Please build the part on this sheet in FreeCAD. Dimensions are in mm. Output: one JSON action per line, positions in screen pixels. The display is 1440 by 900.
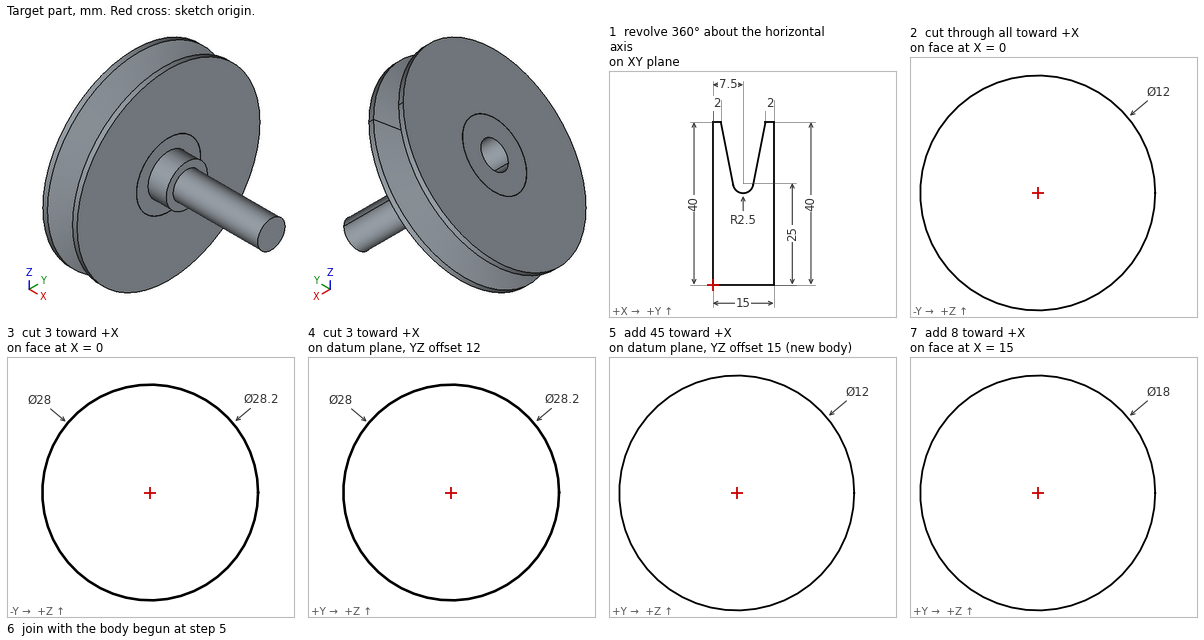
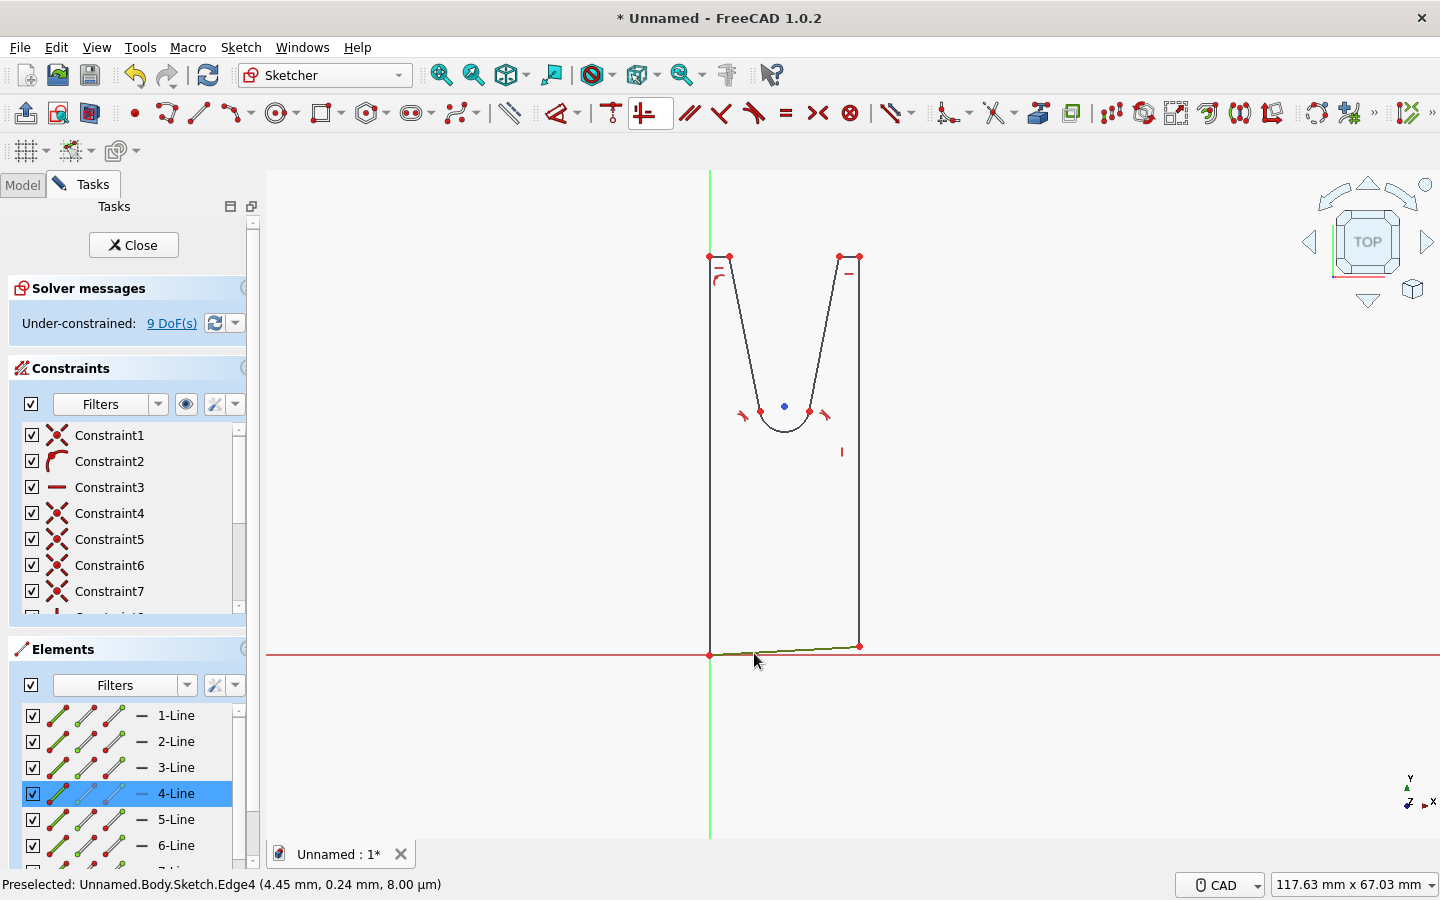
{"action": "key", "text": "h"}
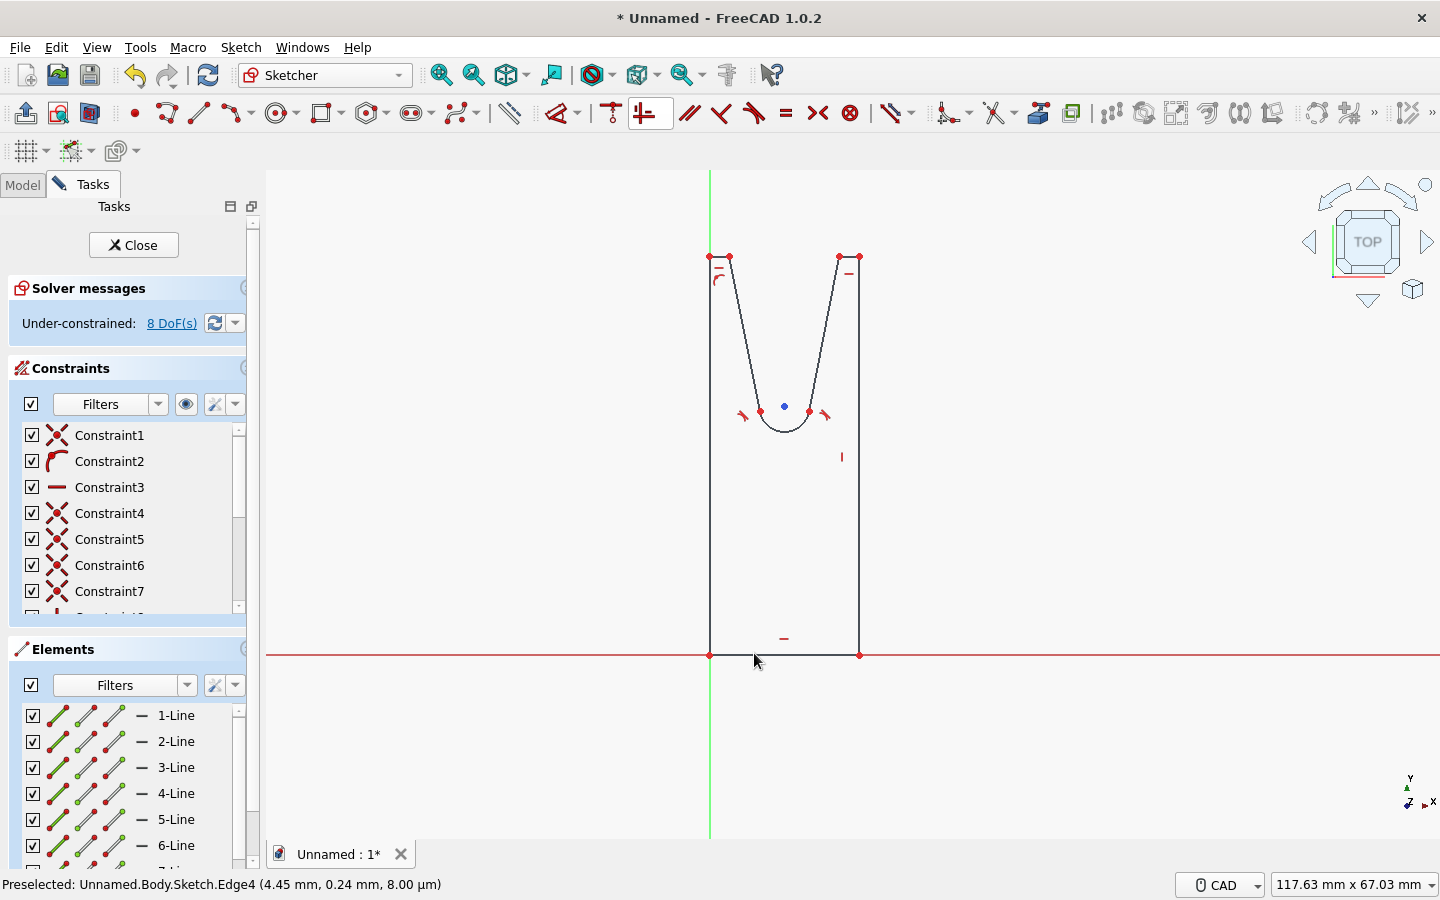
{"action": "scroll", "coordinate": [771, 428], "scroll_direction": "up", "scroll_amount": 3}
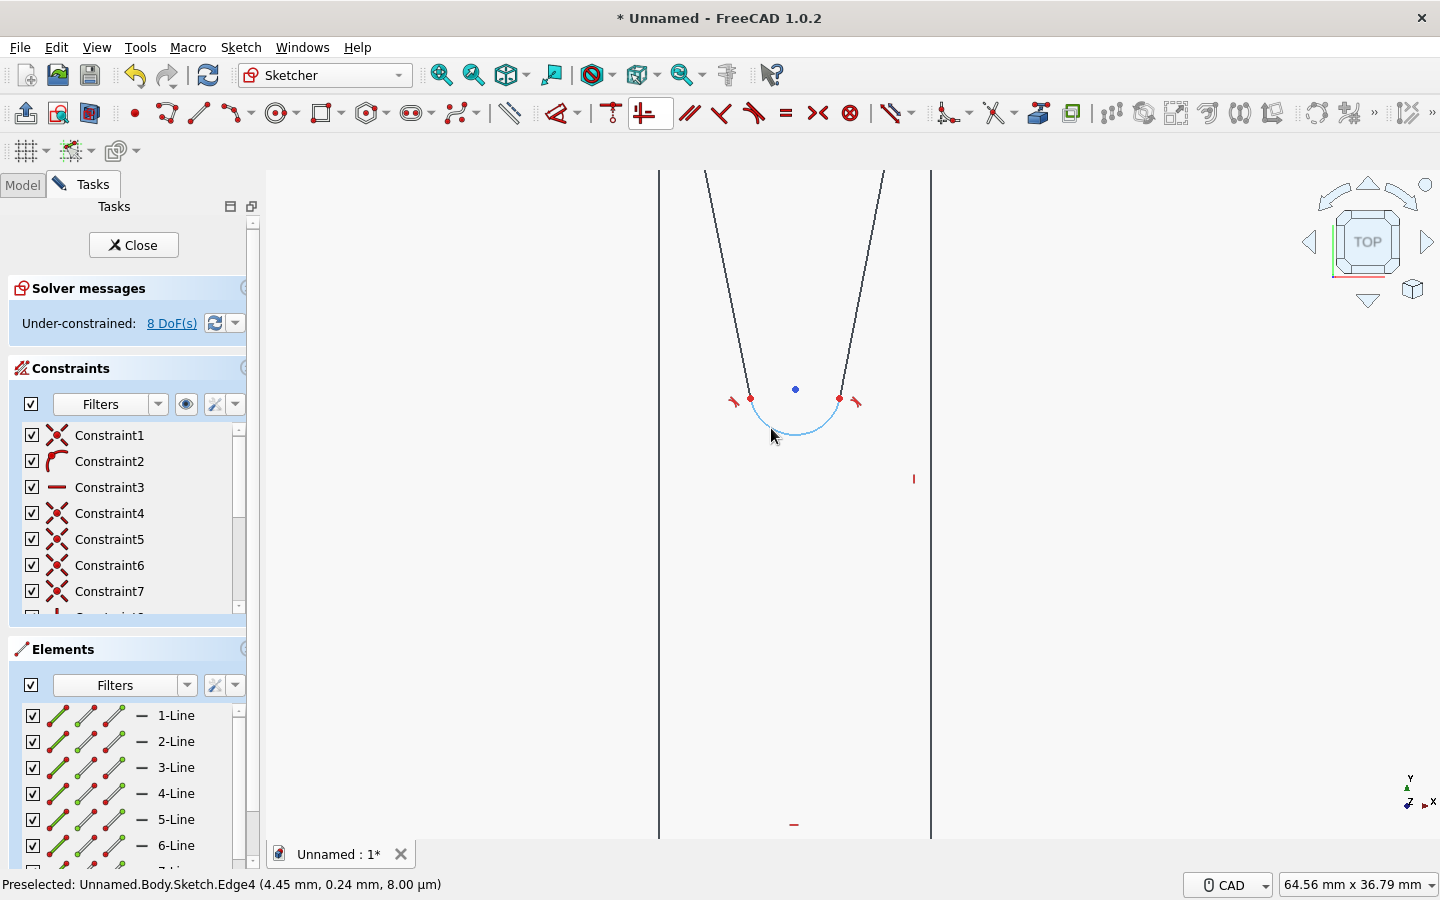
{"action": "left_click", "coordinate": [772, 428]}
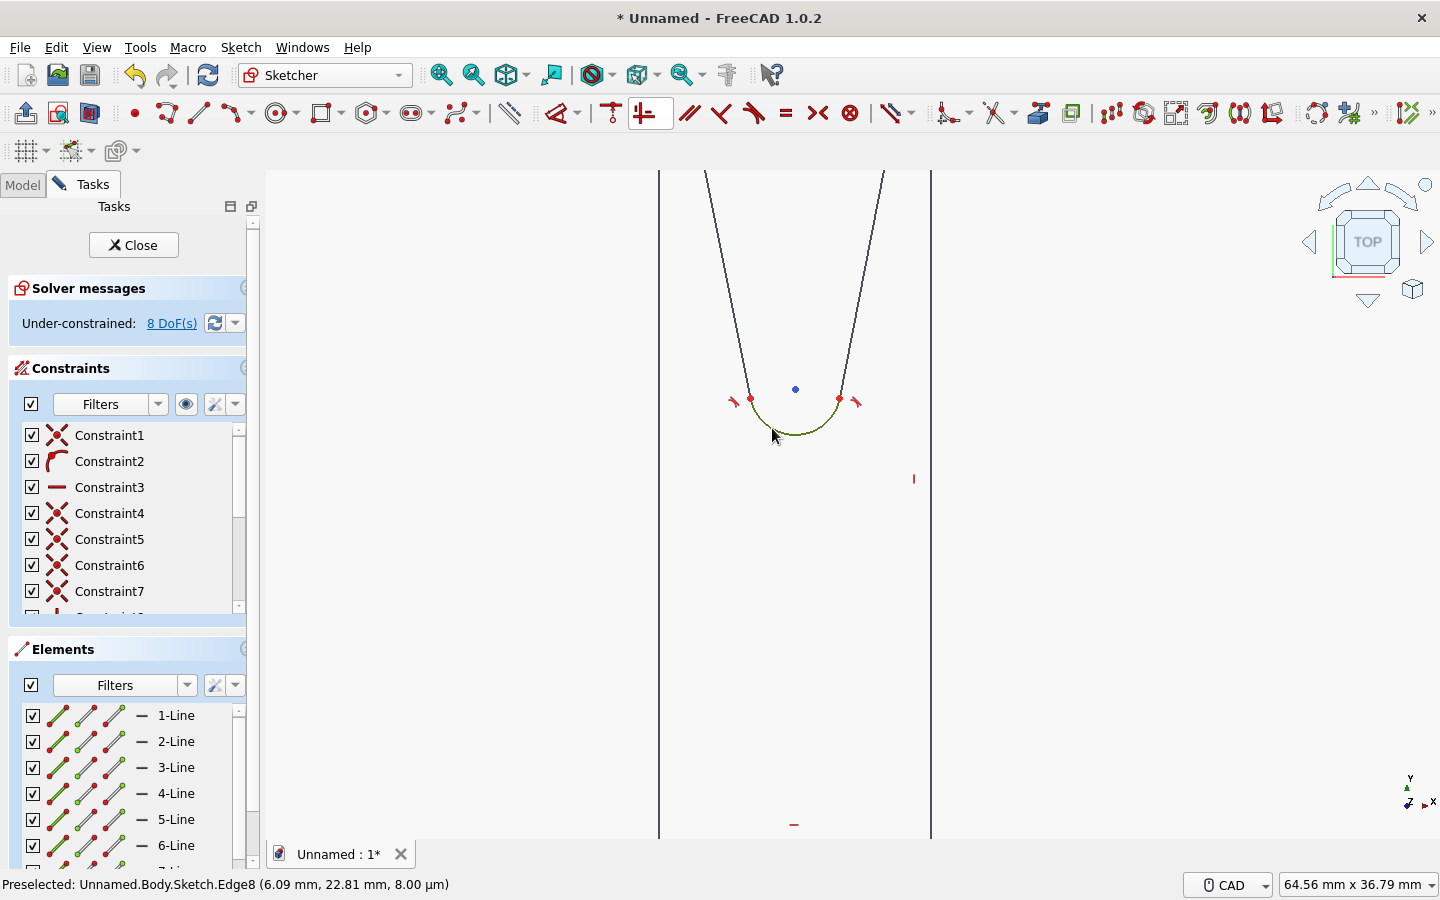
{"action": "left_click", "coordinate": [580, 114]}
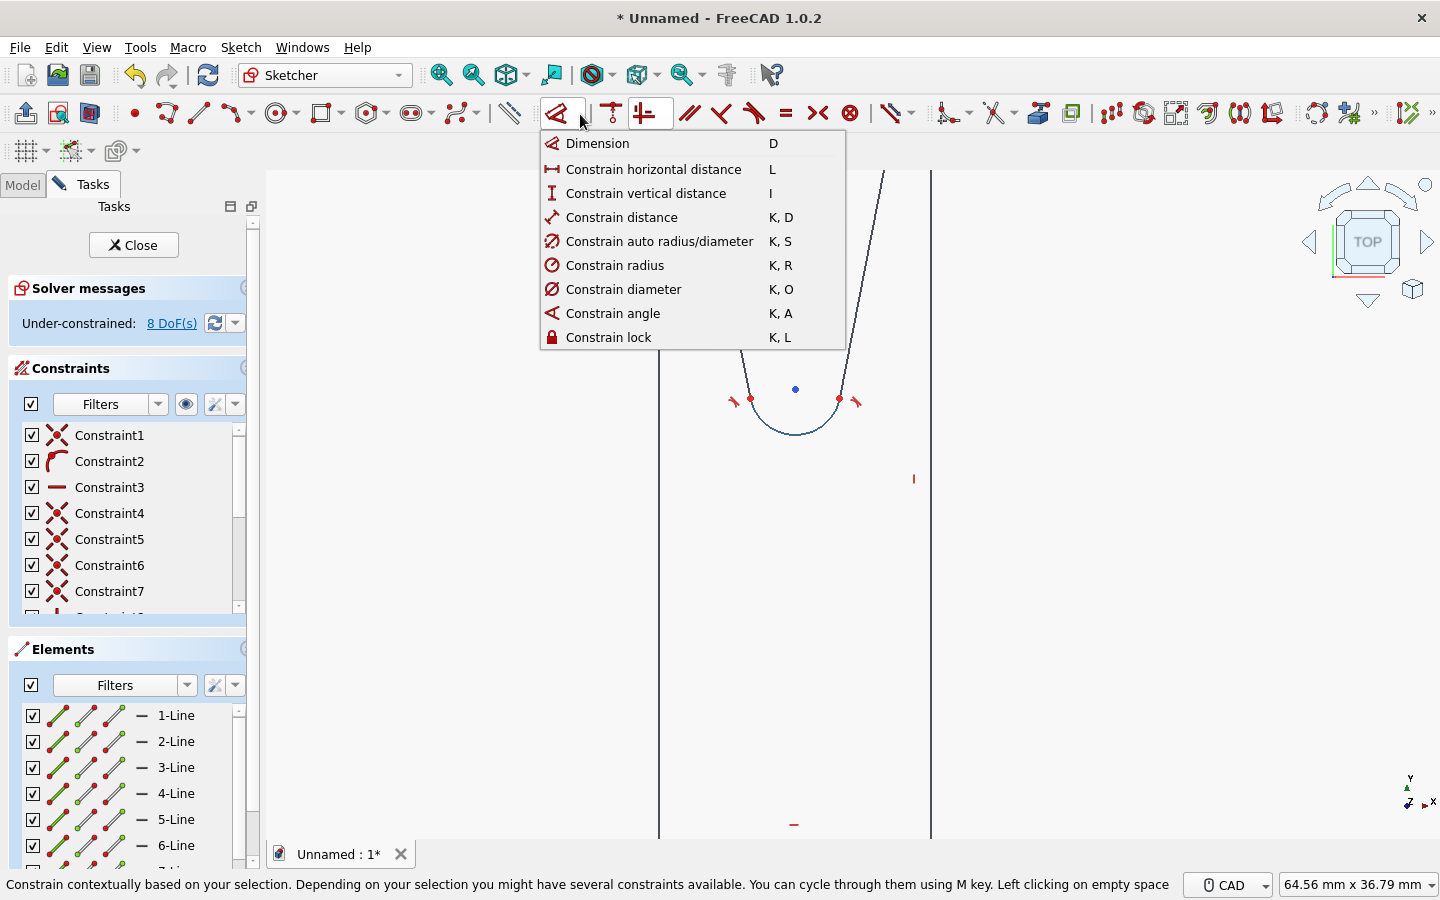
{"action": "left_click", "coordinate": [693, 265]}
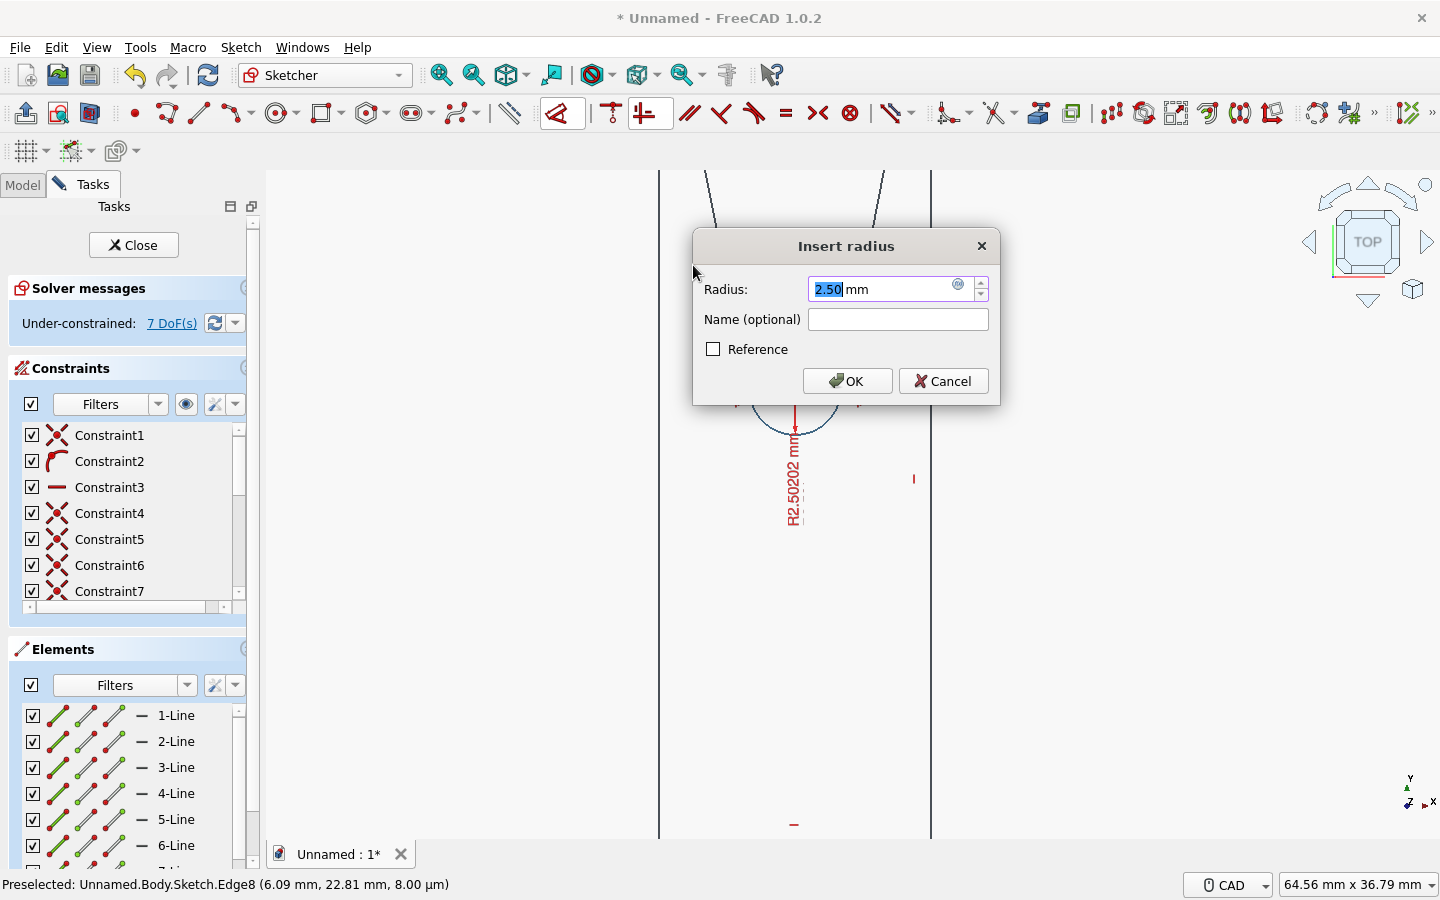
{"action": "type", "text": "2.5"}
{"action": "key", "text": "Return"}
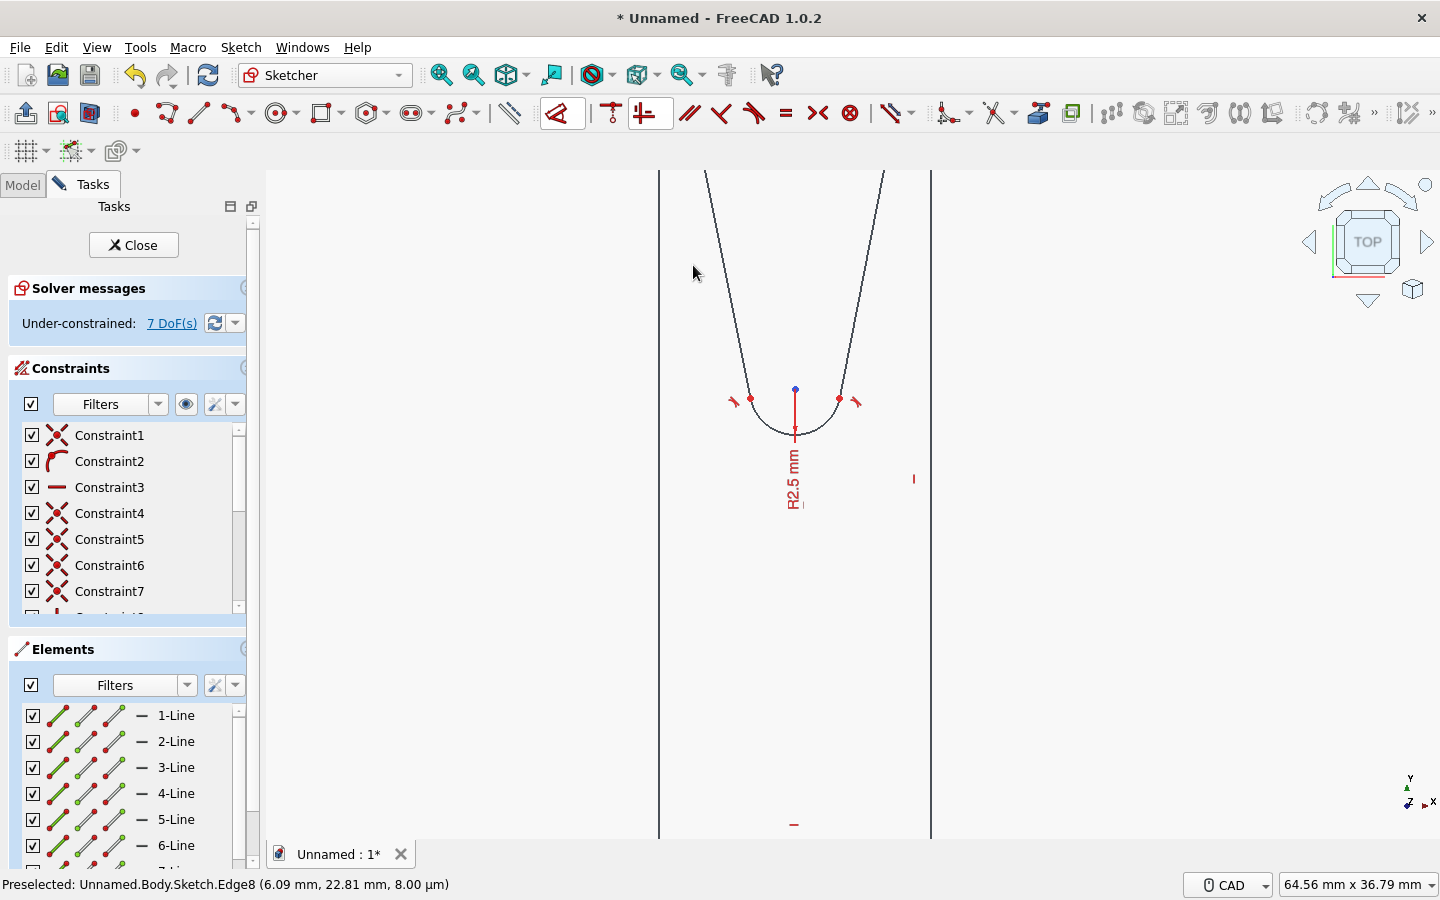
{"action": "scroll", "coordinate": [772, 537], "scroll_direction": "down", "scroll_amount": 3}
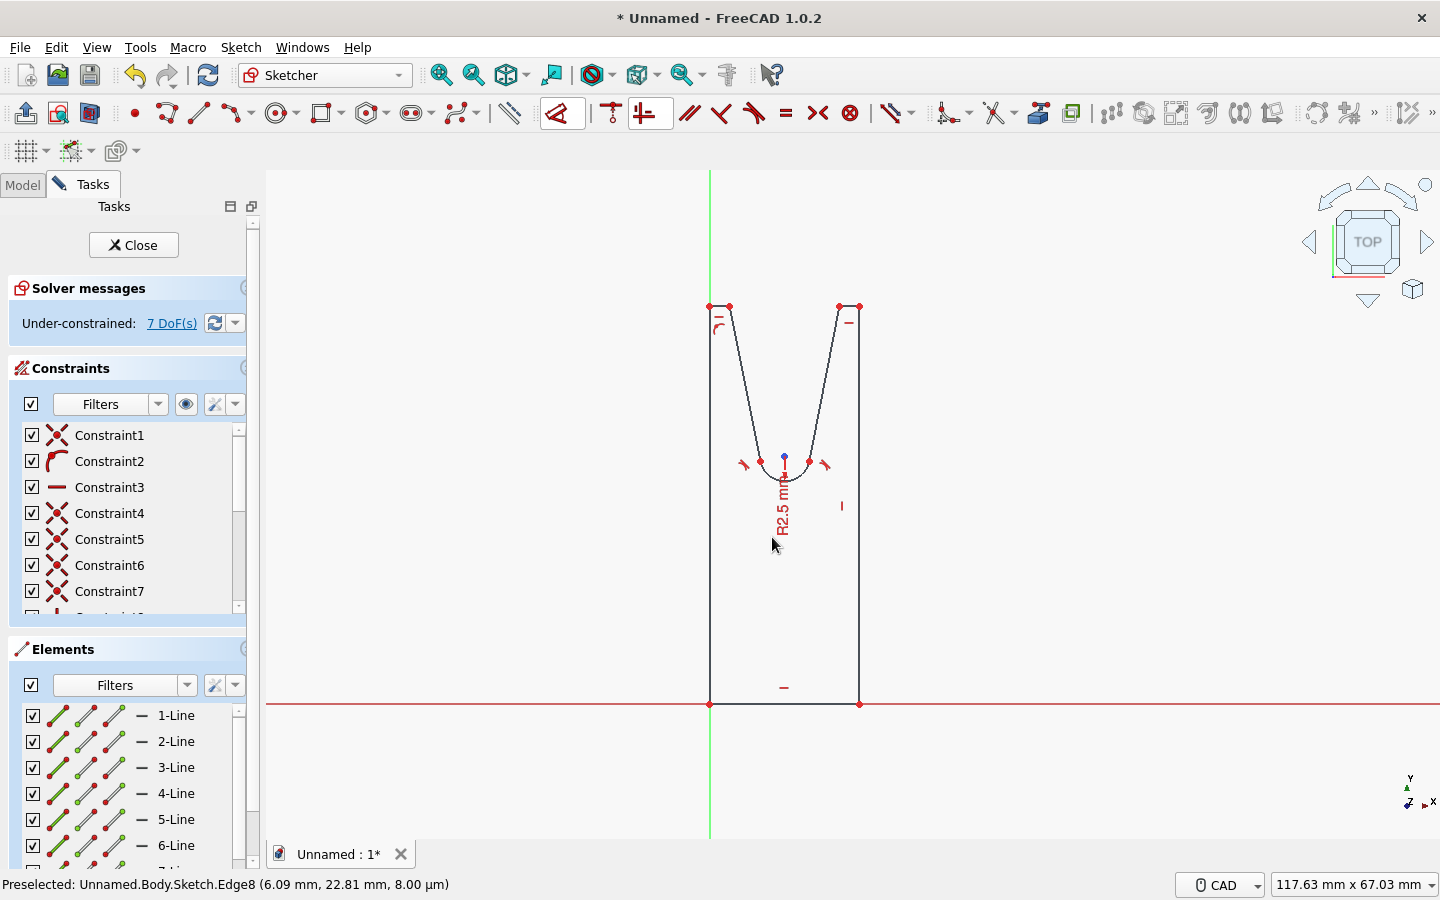
{"action": "scroll", "coordinate": [724, 306], "scroll_direction": "up", "scroll_amount": 5}